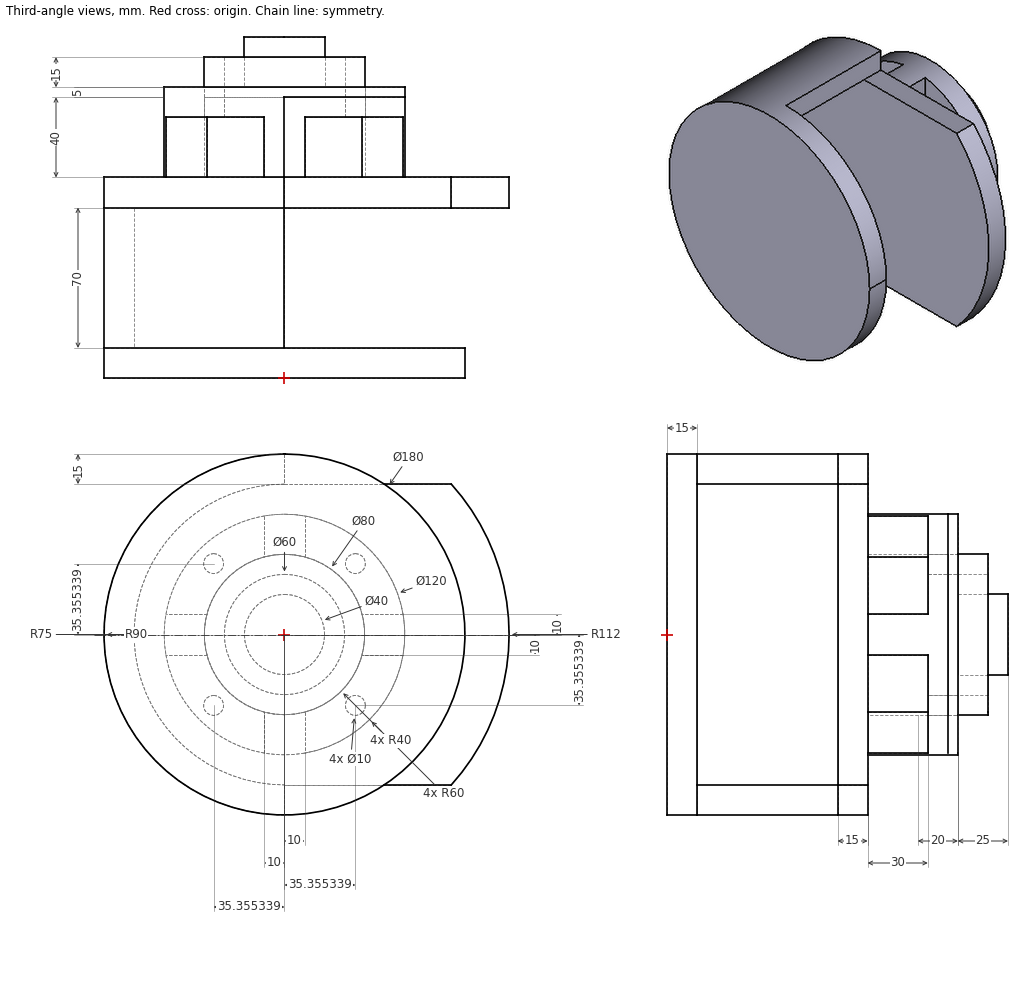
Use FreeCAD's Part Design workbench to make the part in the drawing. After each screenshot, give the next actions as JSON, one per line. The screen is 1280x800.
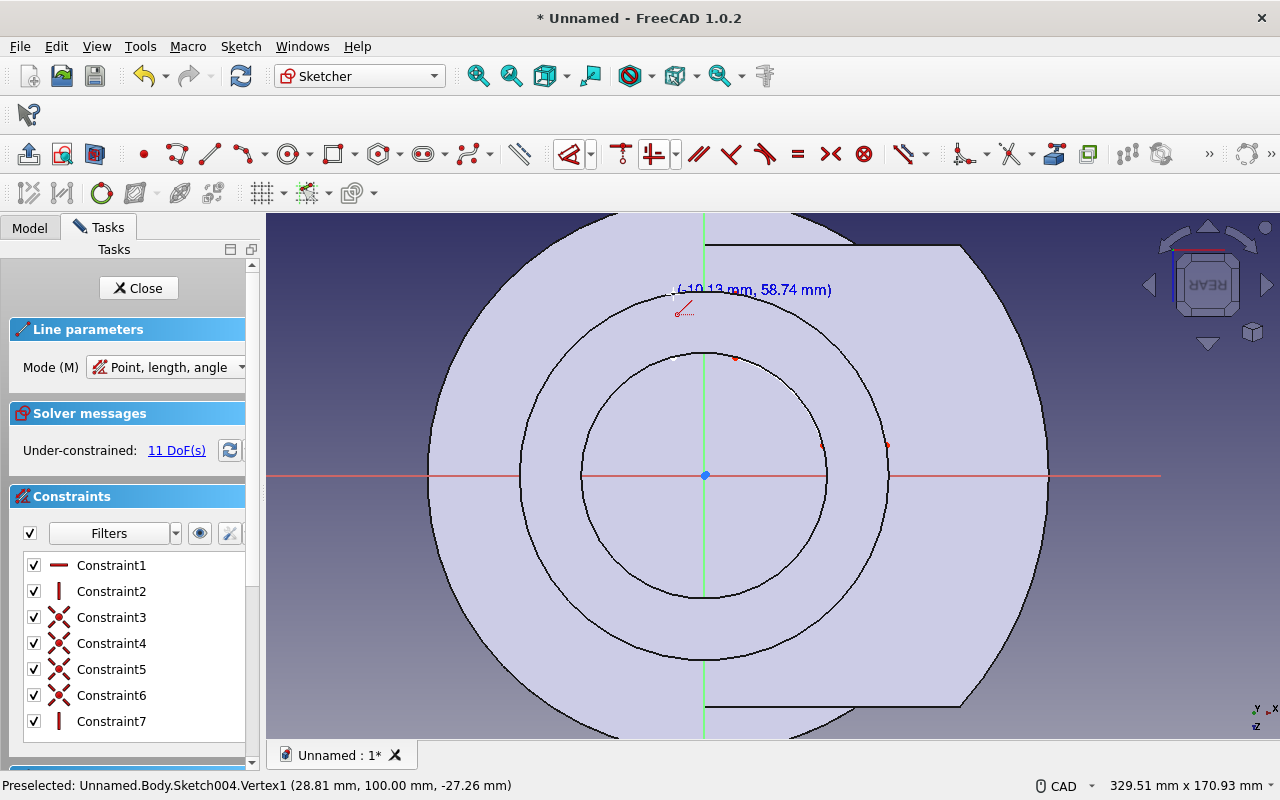
{"action": "left_click", "coordinate": [522, 445]}
{"action": "left_click", "coordinate": [585, 445]}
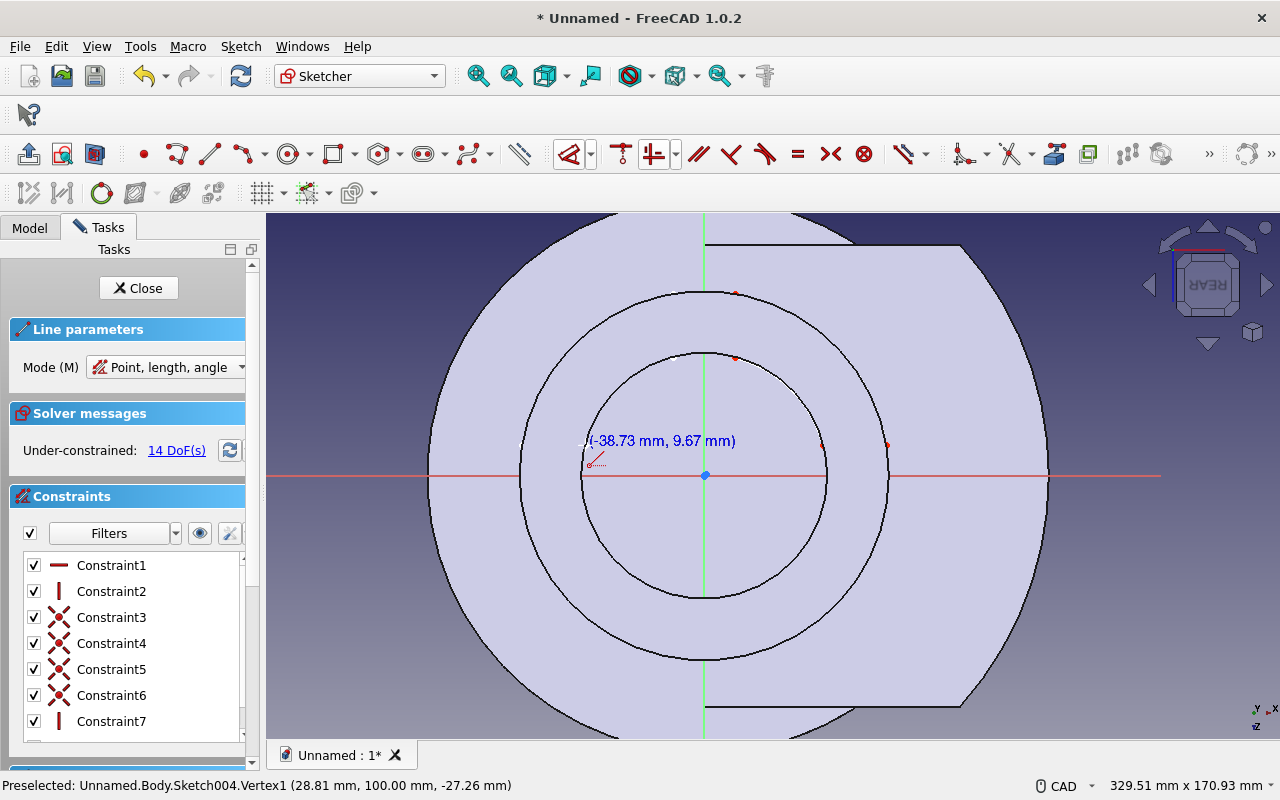
{"action": "left_click", "coordinate": [242, 154]}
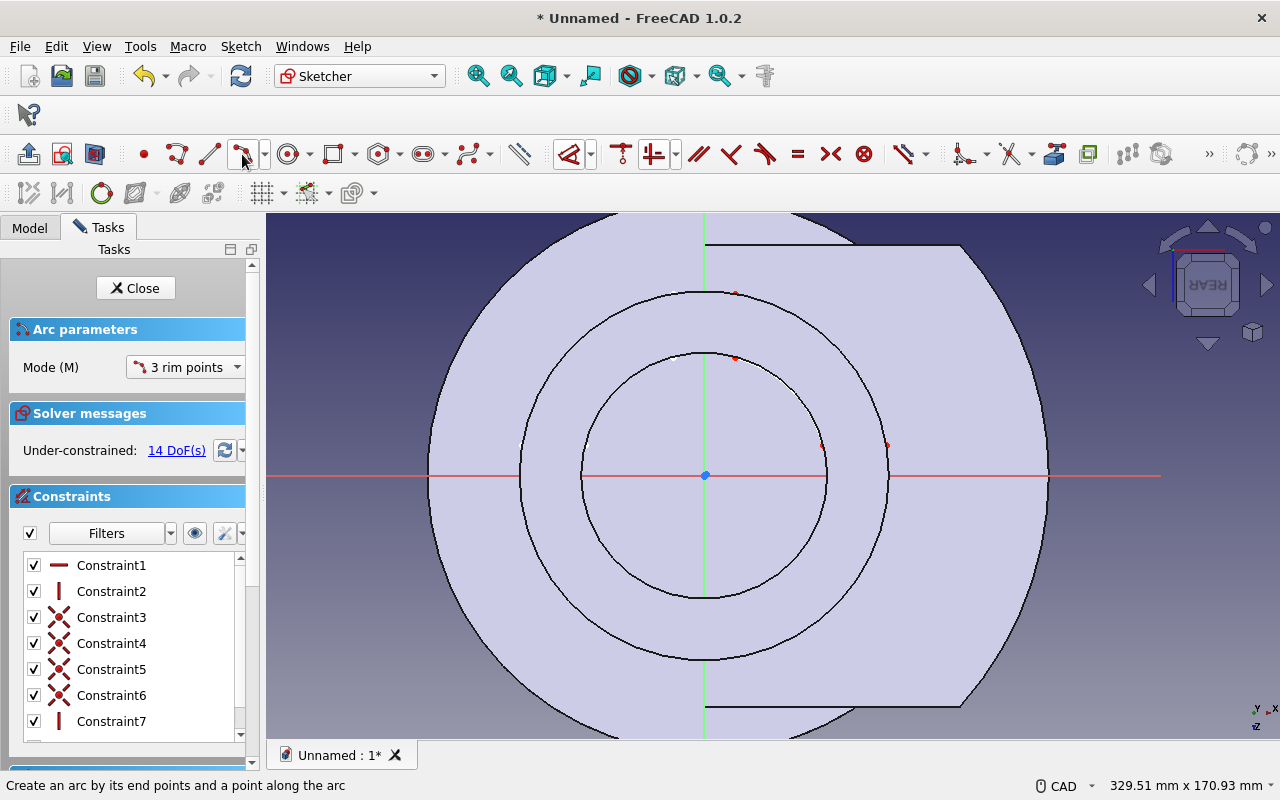
{"action": "left_click", "coordinate": [673, 295]}
{"action": "left_click", "coordinate": [522, 446]}
{"action": "left_click", "coordinate": [574, 345]}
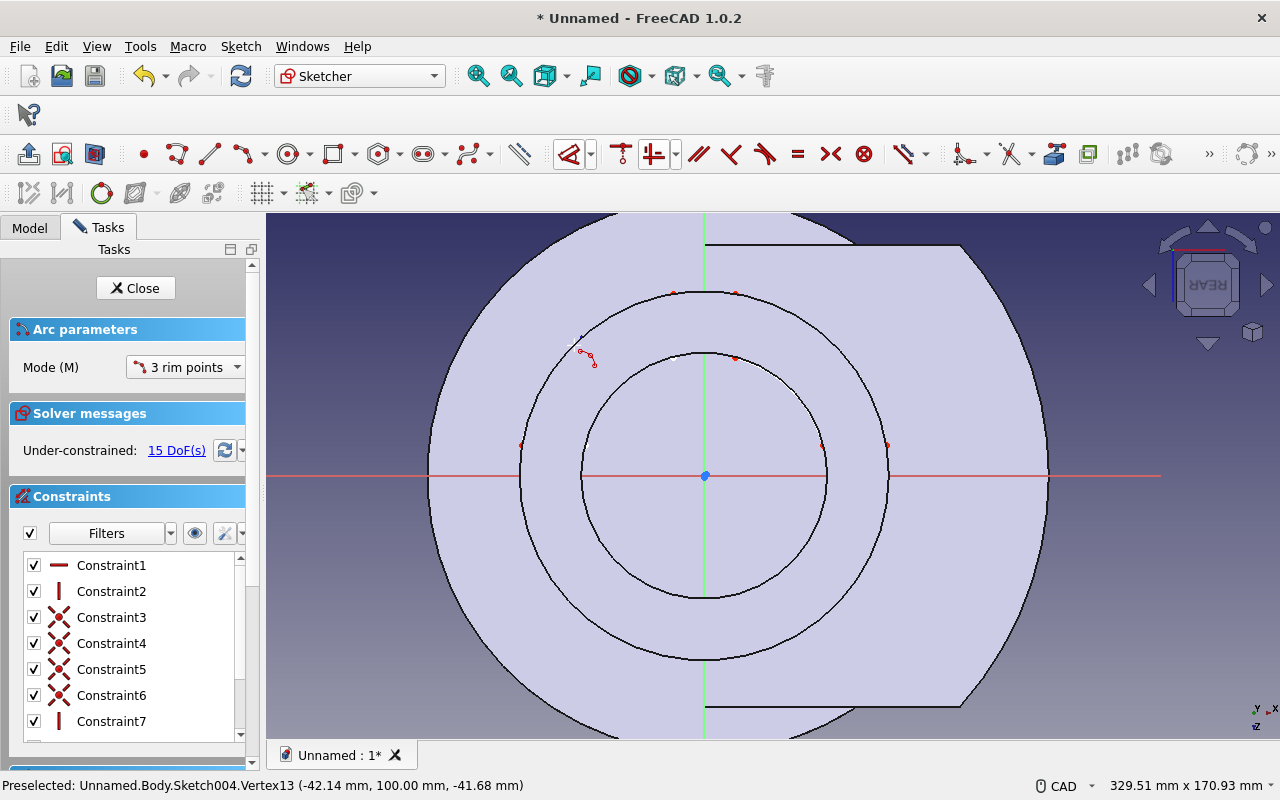
{"action": "left_click", "coordinate": [585, 446]}
{"action": "left_click", "coordinate": [673, 358]}
{"action": "left_click", "coordinate": [617, 389]}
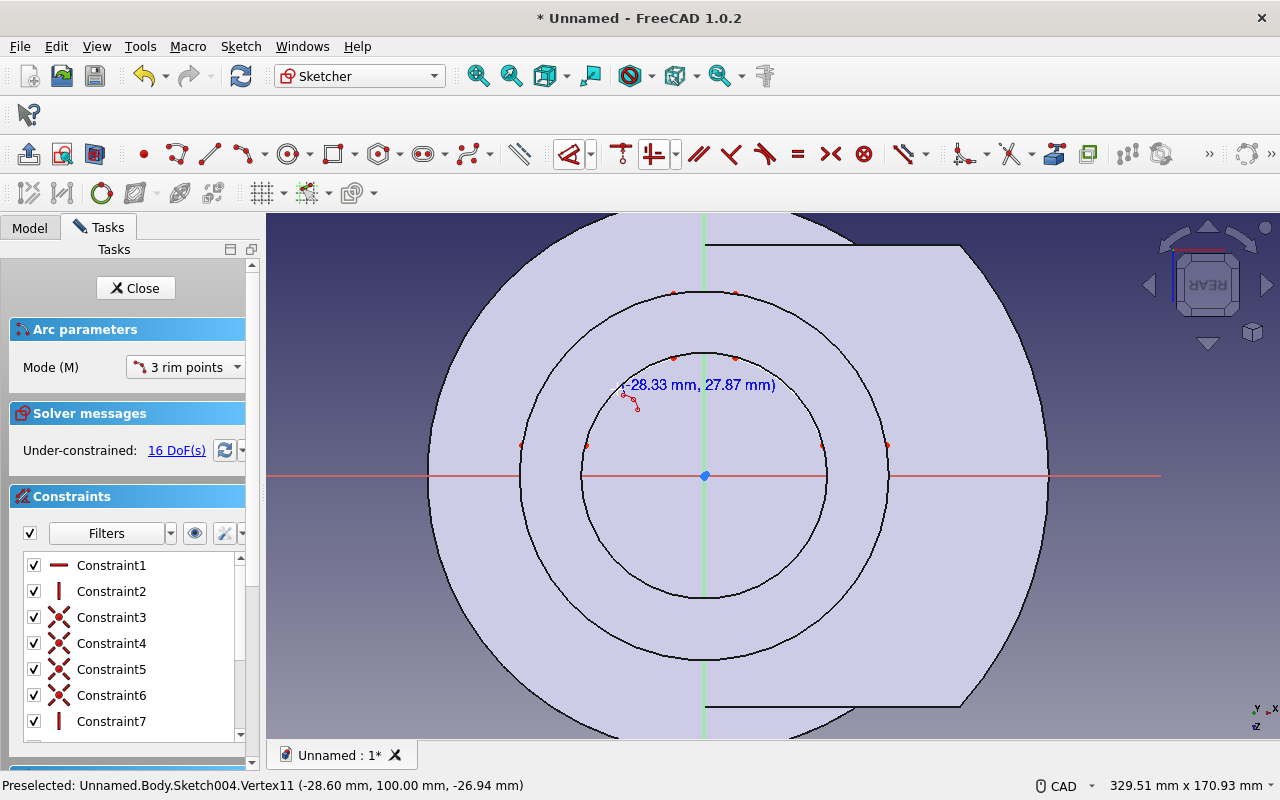
{"action": "left_click", "coordinate": [210, 154]}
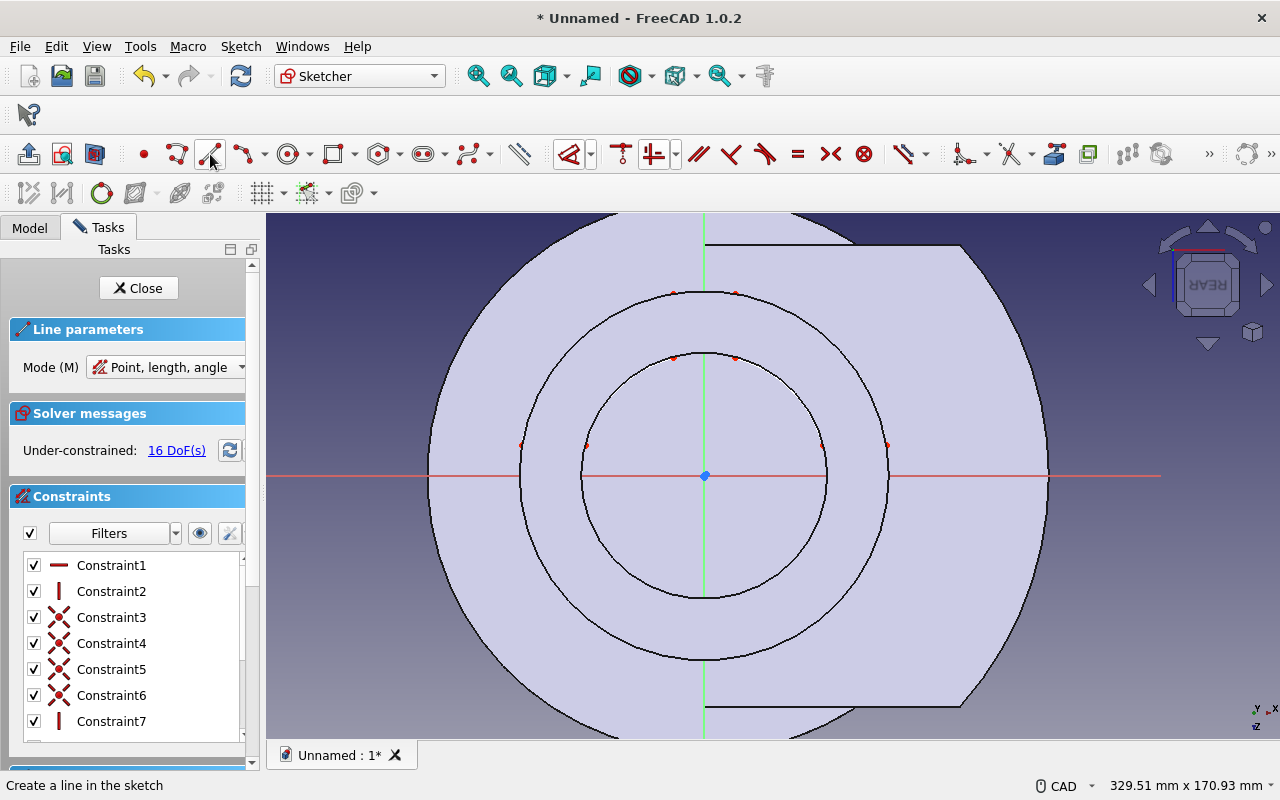
{"action": "left_click", "coordinate": [886, 507]}
{"action": "left_click", "coordinate": [823, 507]}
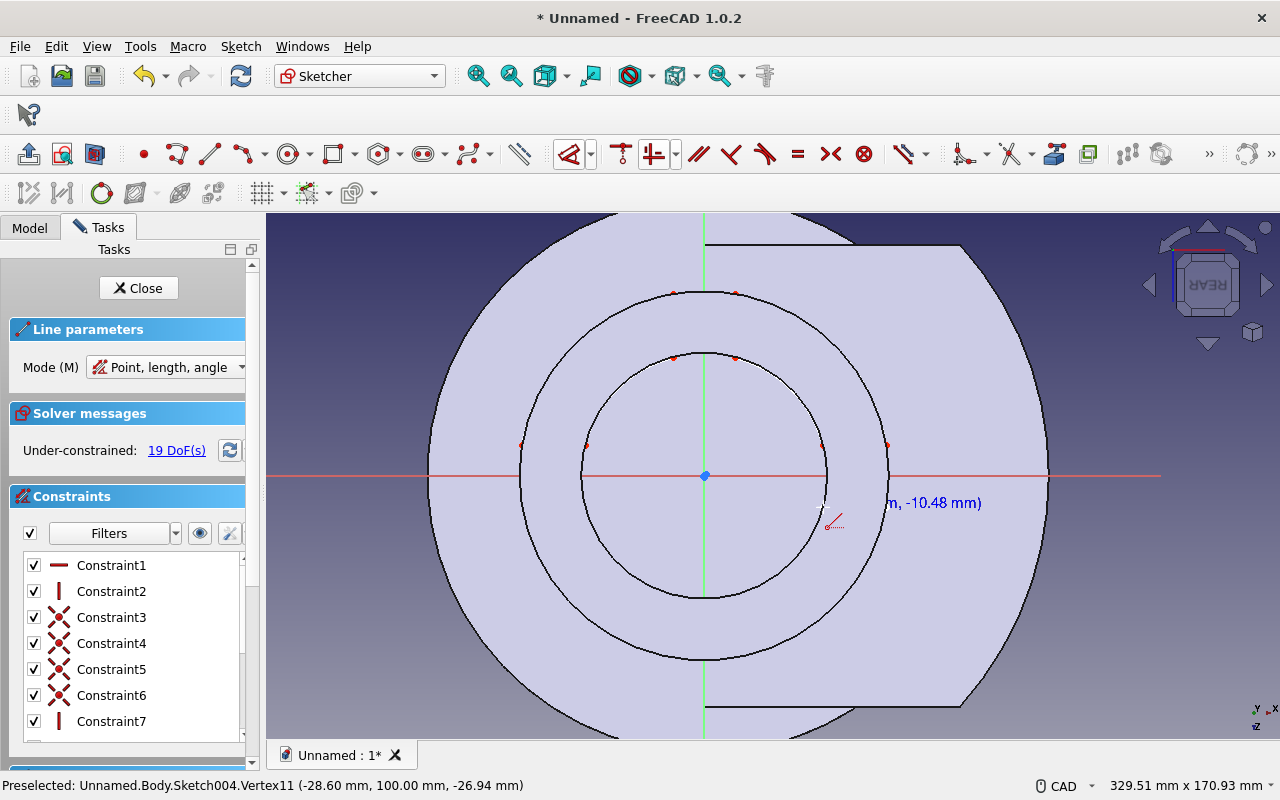
{"action": "left_click", "coordinate": [735, 595]}
{"action": "left_click", "coordinate": [735, 658]}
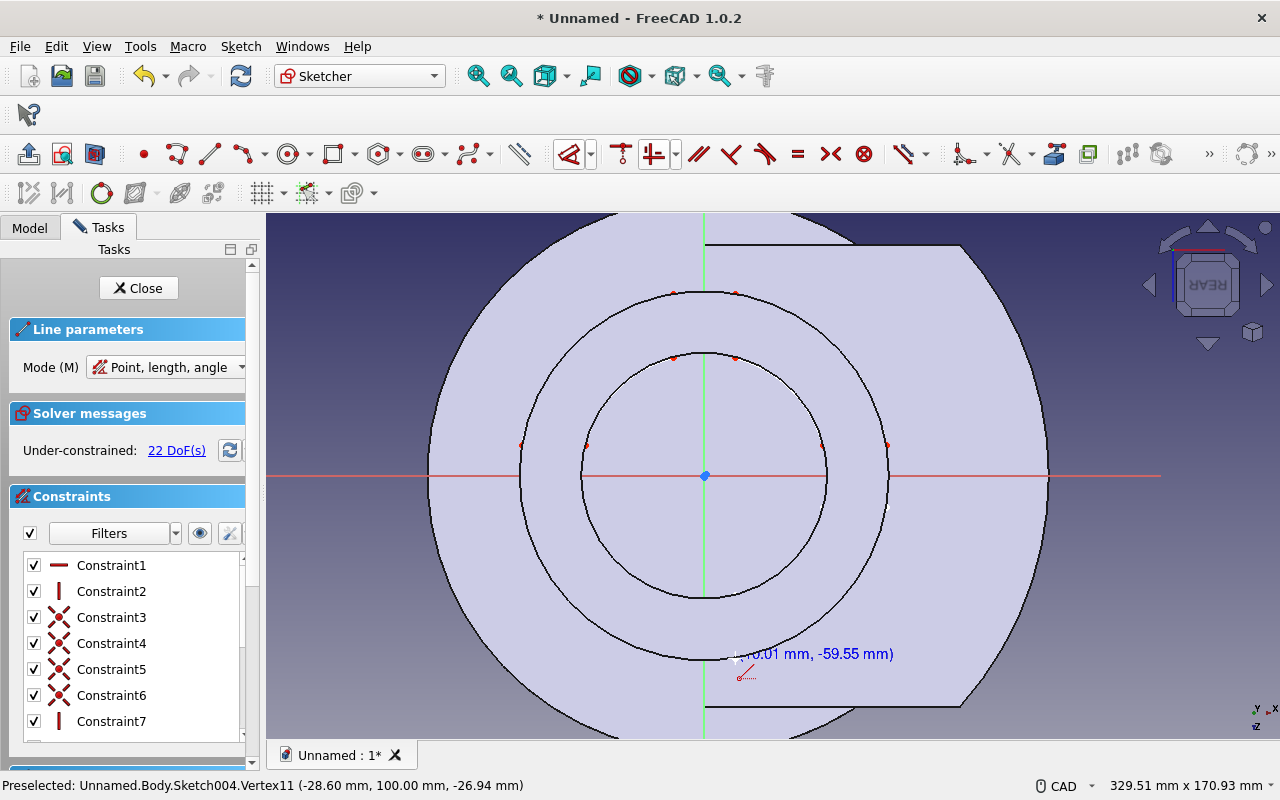
{"action": "left_click", "coordinate": [242, 154]}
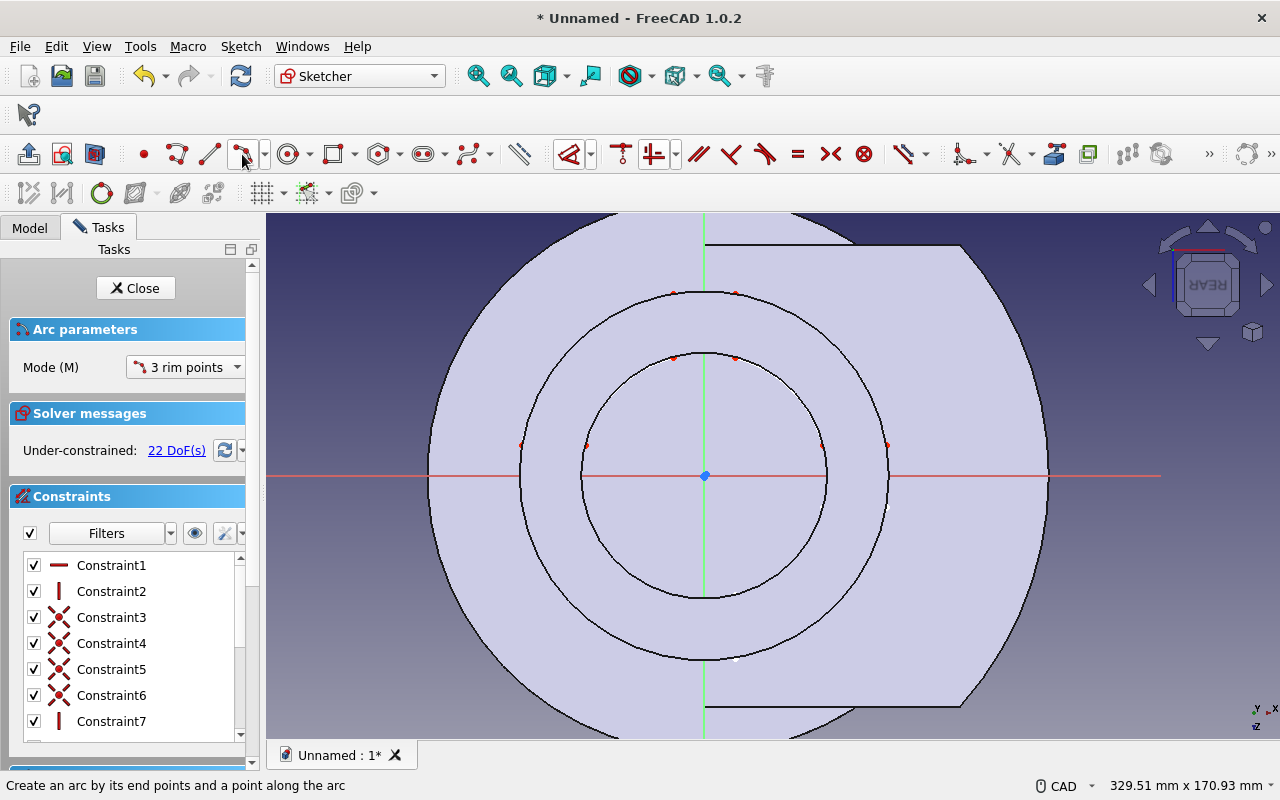
{"action": "left_click", "coordinate": [823, 508]}
{"action": "left_click", "coordinate": [735, 596]}
{"action": "left_click", "coordinate": [791, 563]}